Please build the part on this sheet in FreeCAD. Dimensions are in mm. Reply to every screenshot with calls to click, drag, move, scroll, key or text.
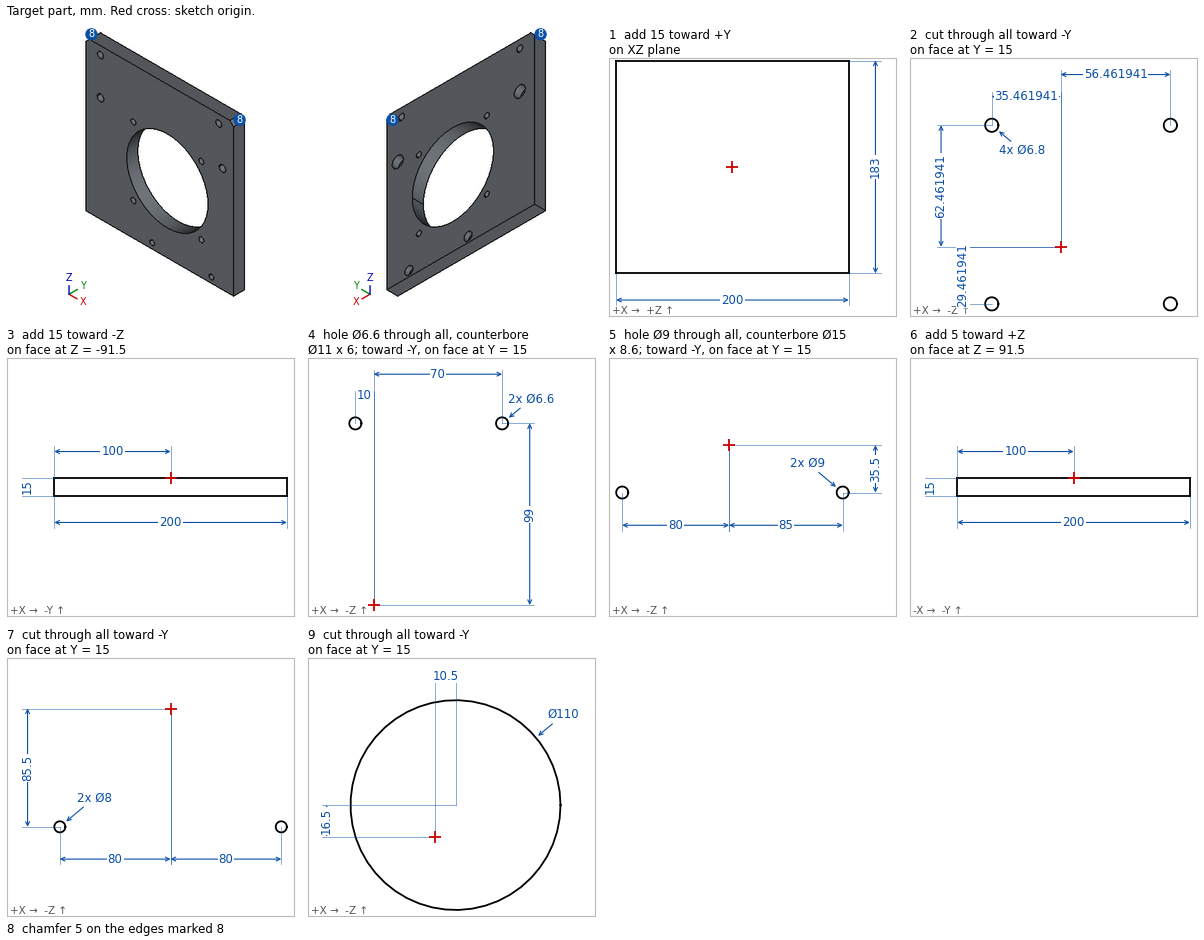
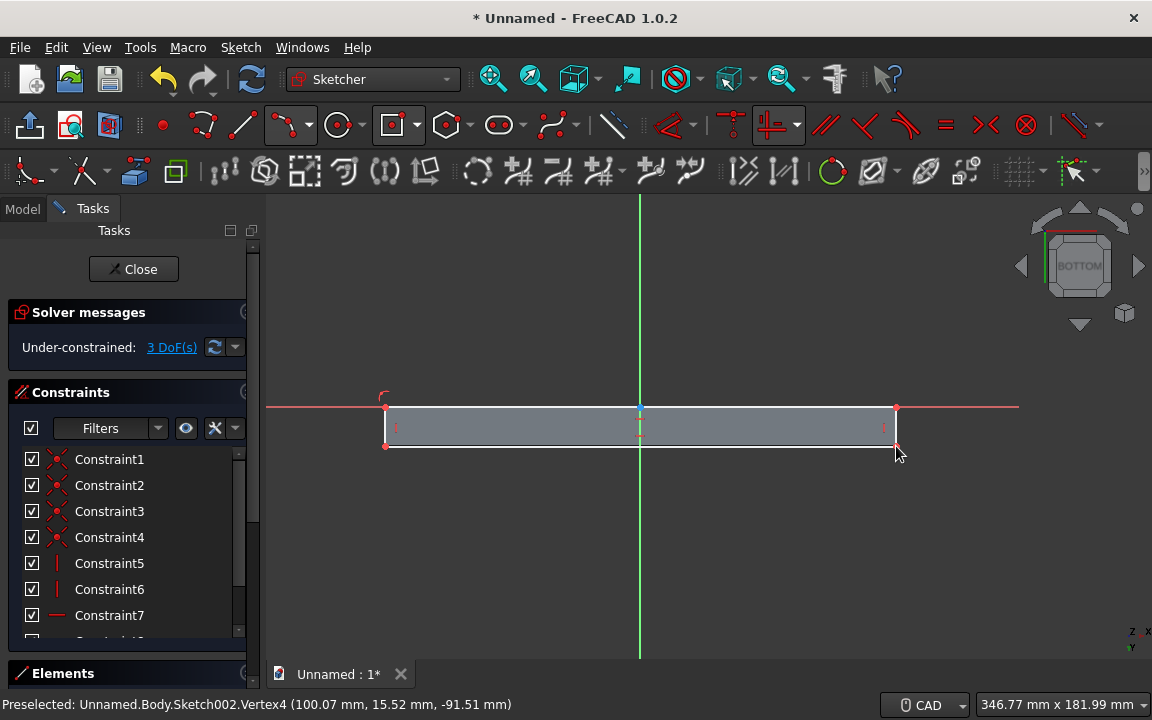
click(668, 126)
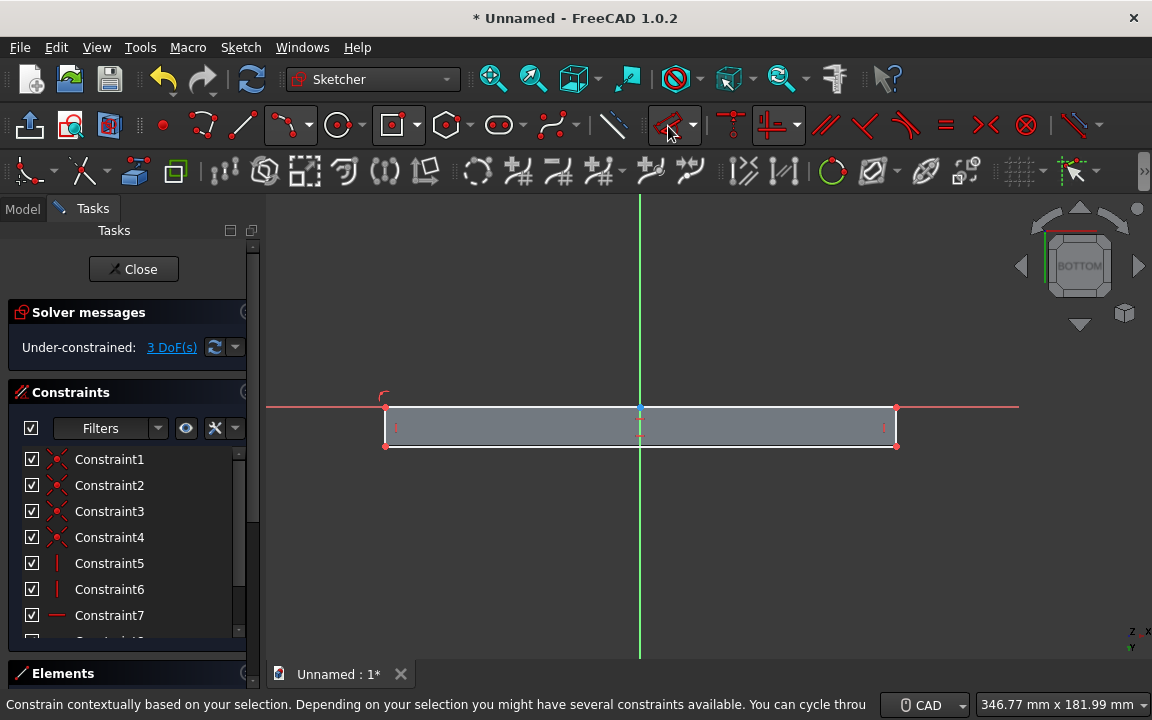
click(385, 419)
click(351, 427)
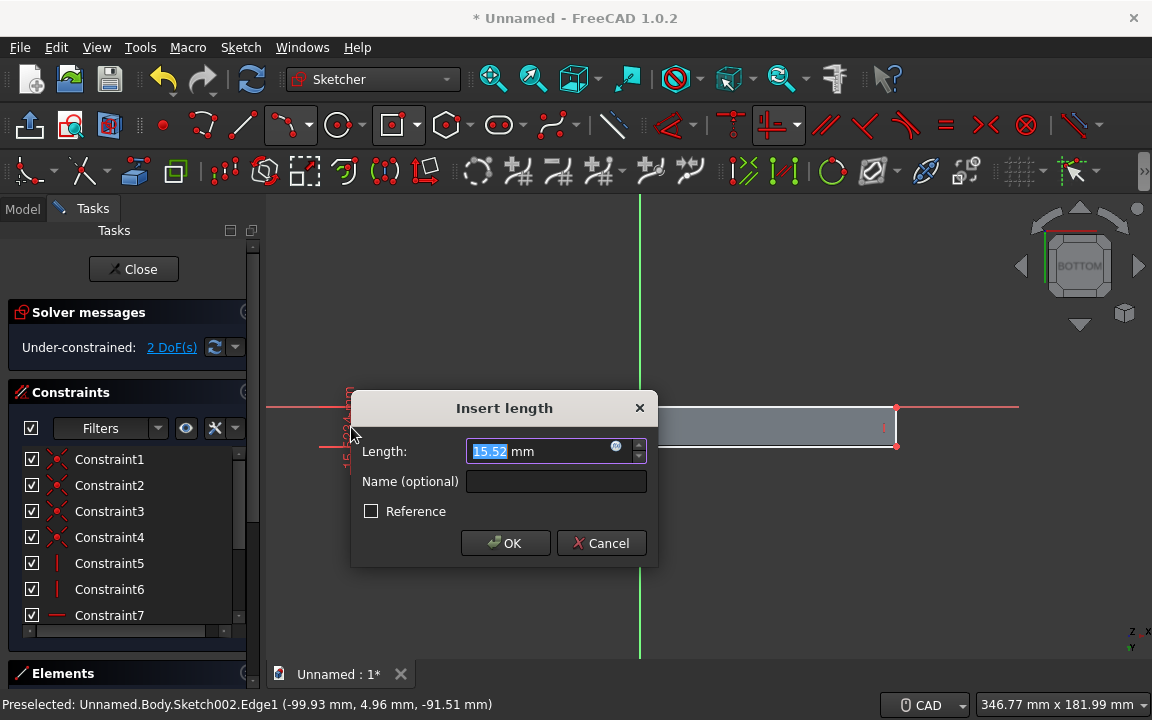
text(15)
key(Return)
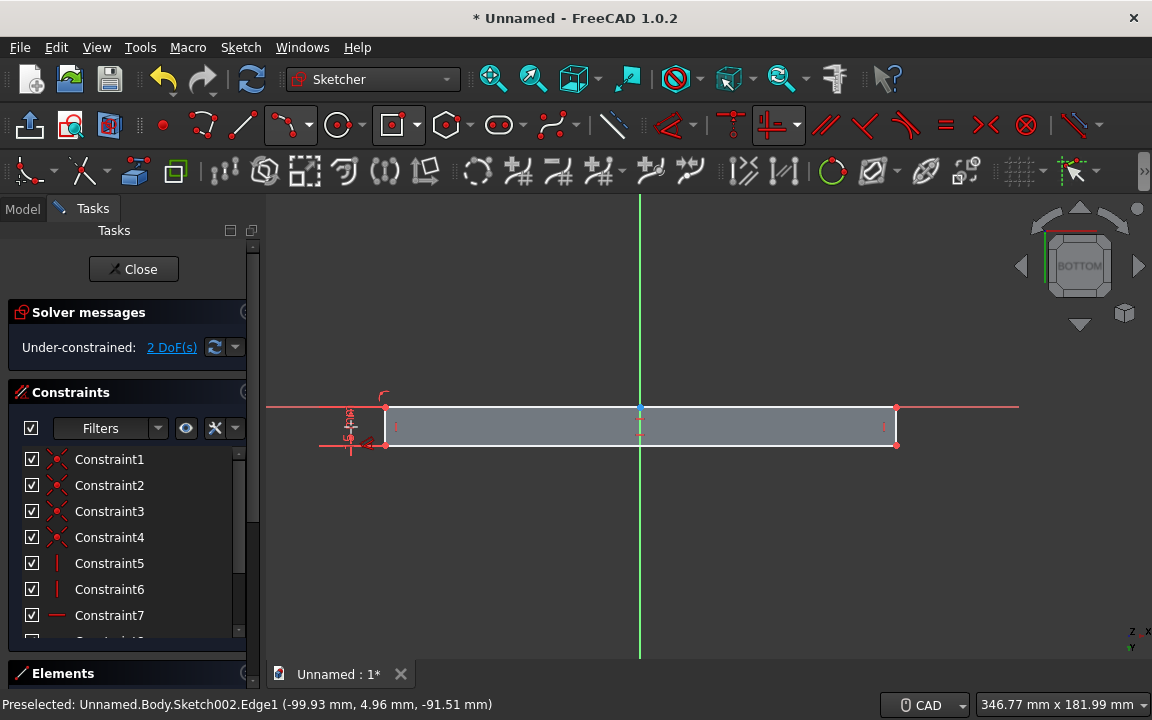
click(538, 446)
click(523, 480)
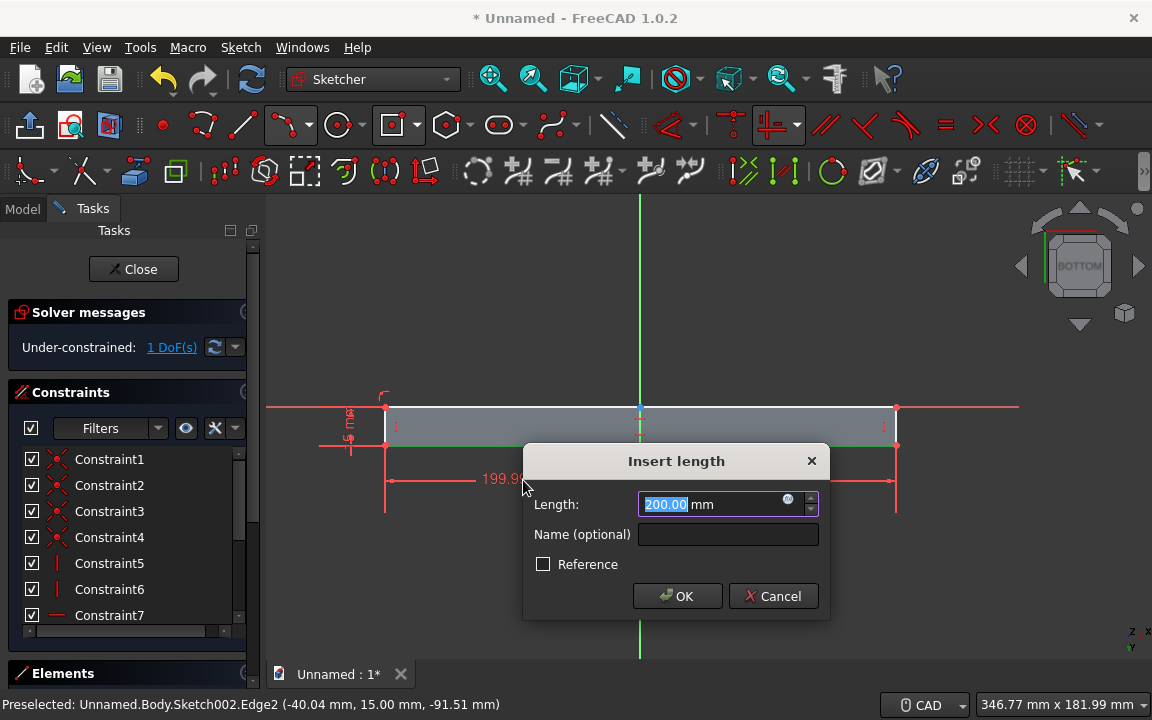
text(200)
key(Return)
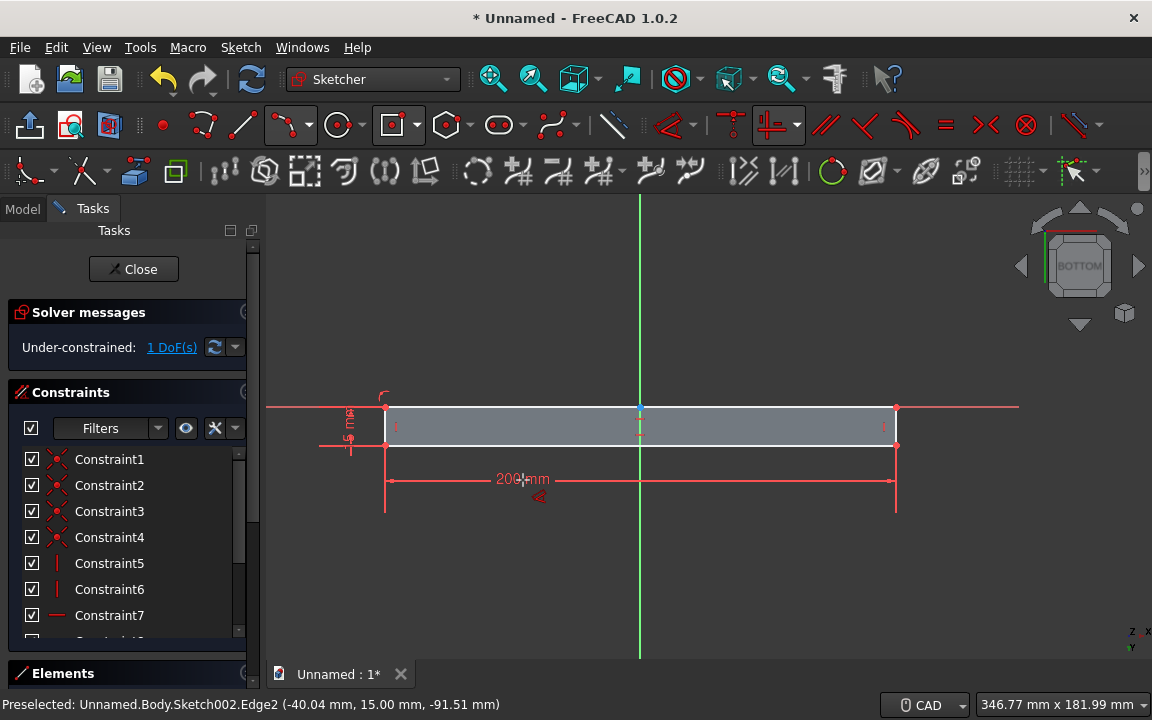
click(385, 407)
click(513, 373)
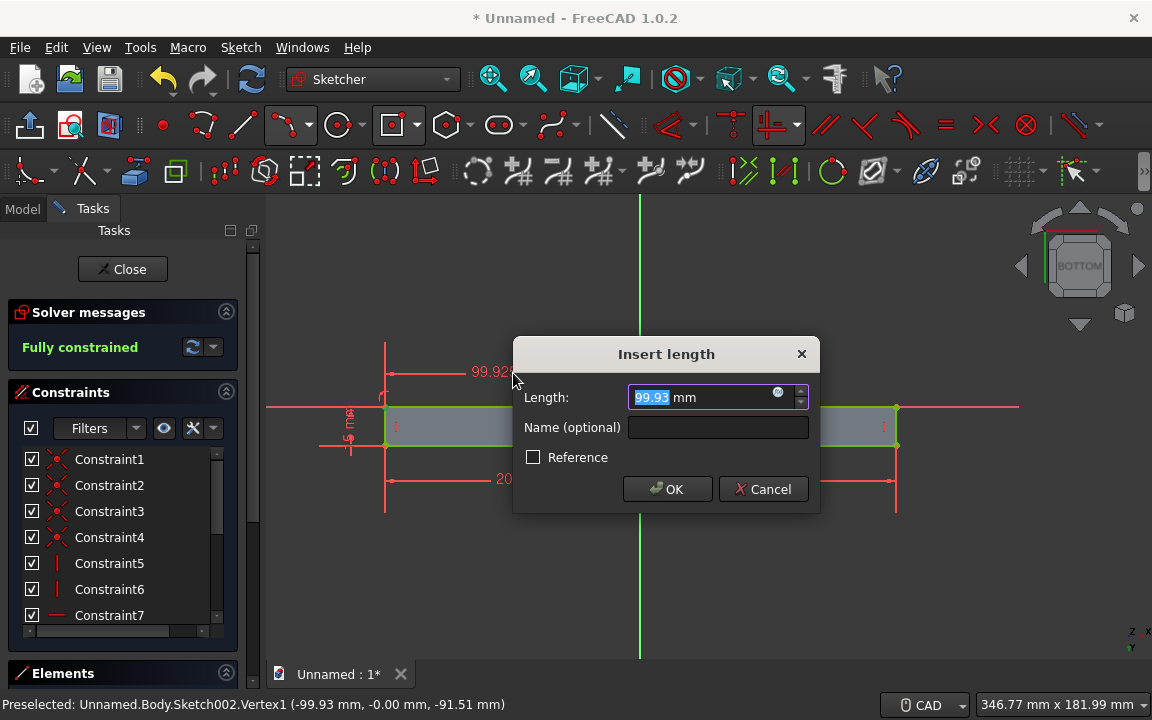
text(100)
key(Return)
key(Escape)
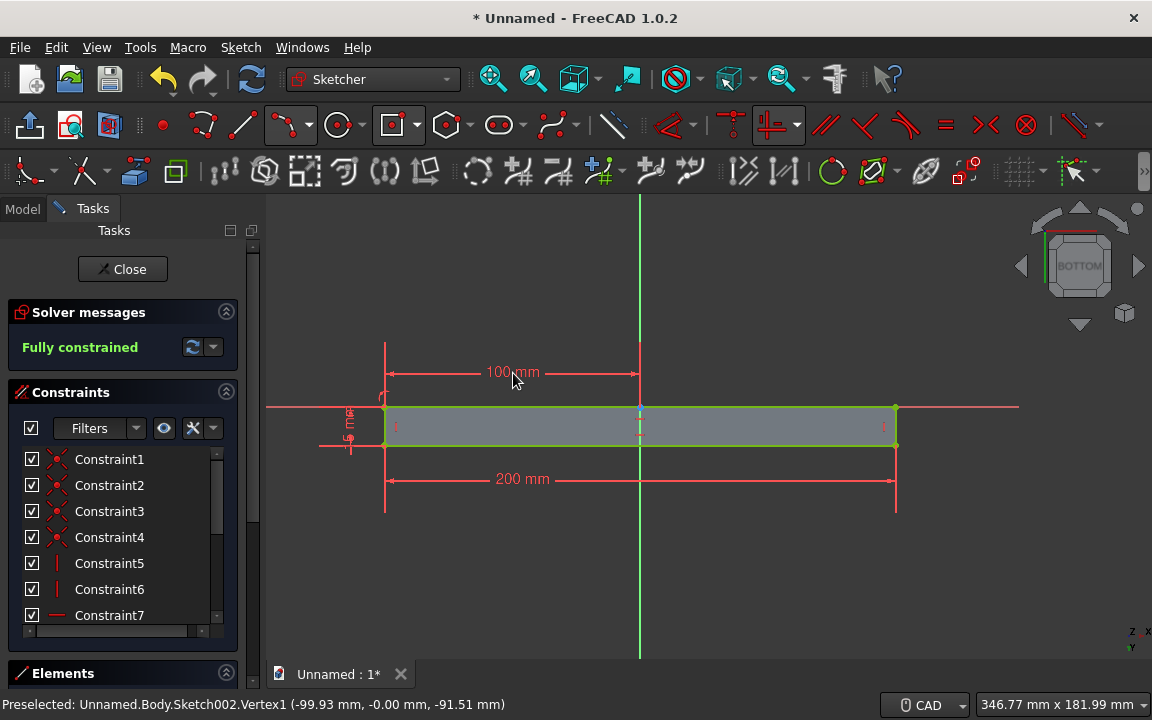
click(123, 269)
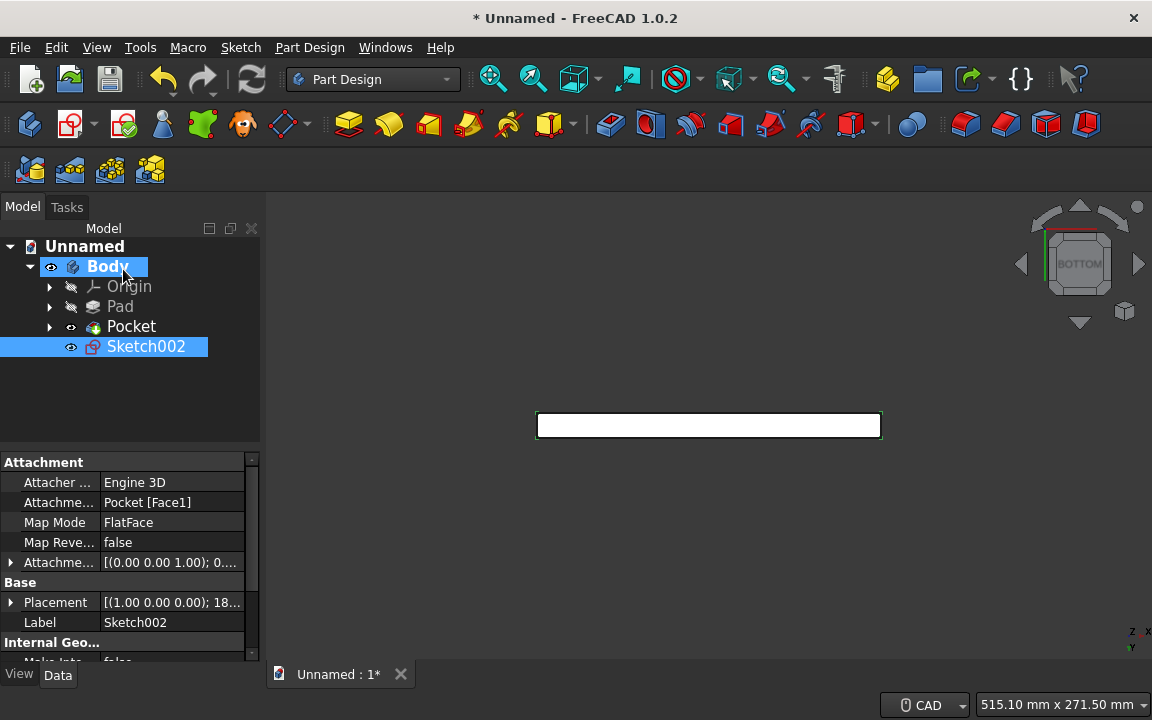
click(350, 124)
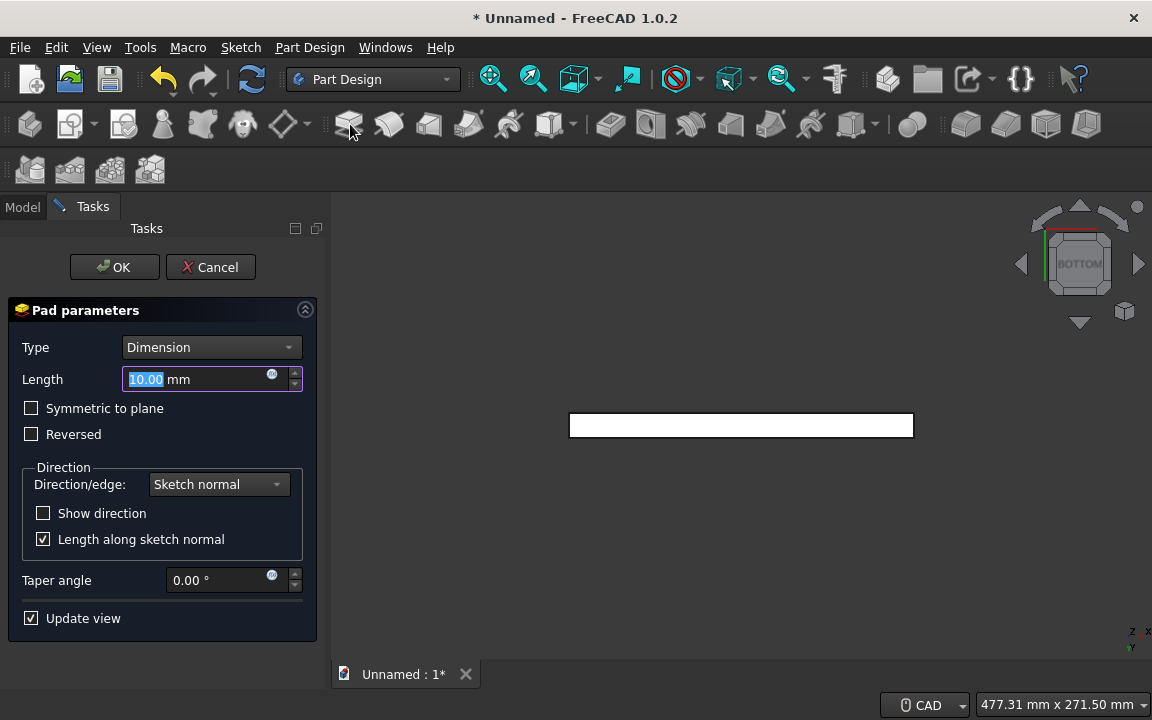
text(15)
key(Tab)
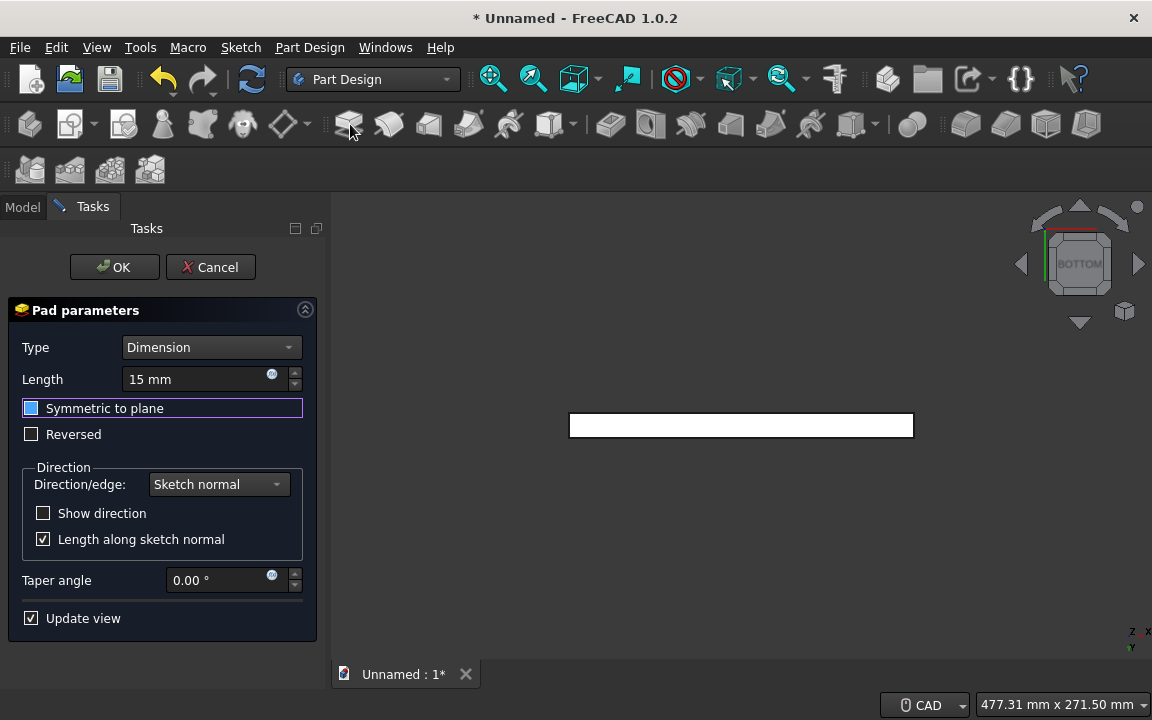
click(115, 267)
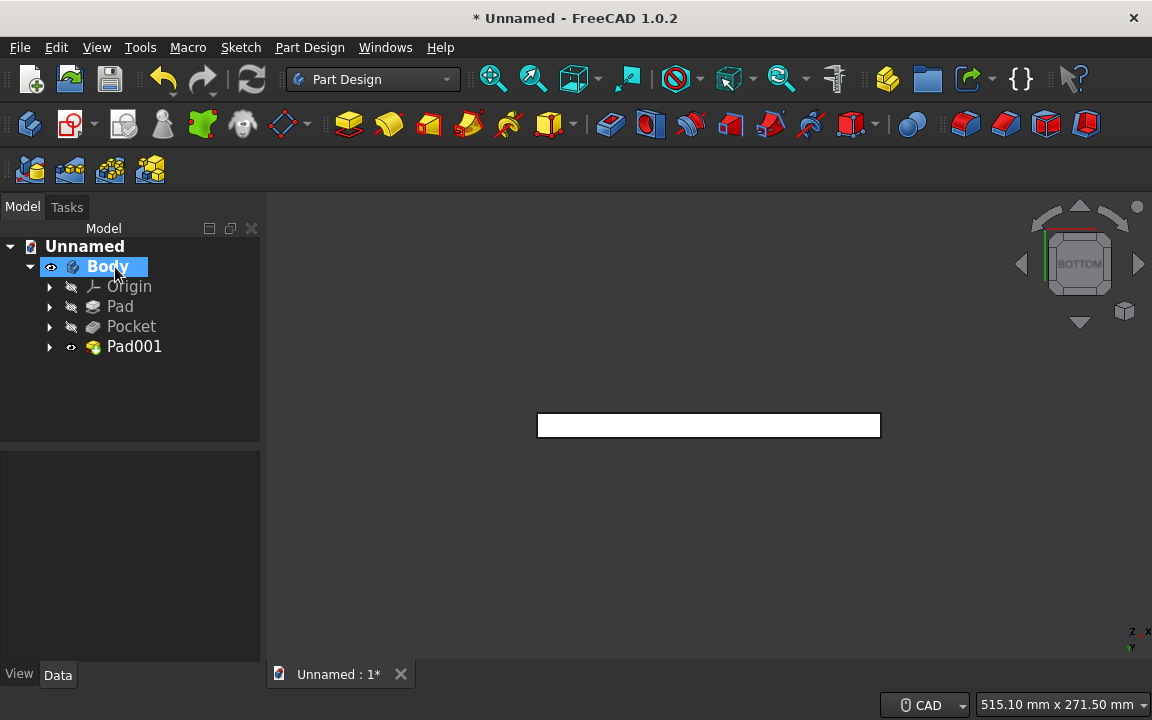
click(494, 80)